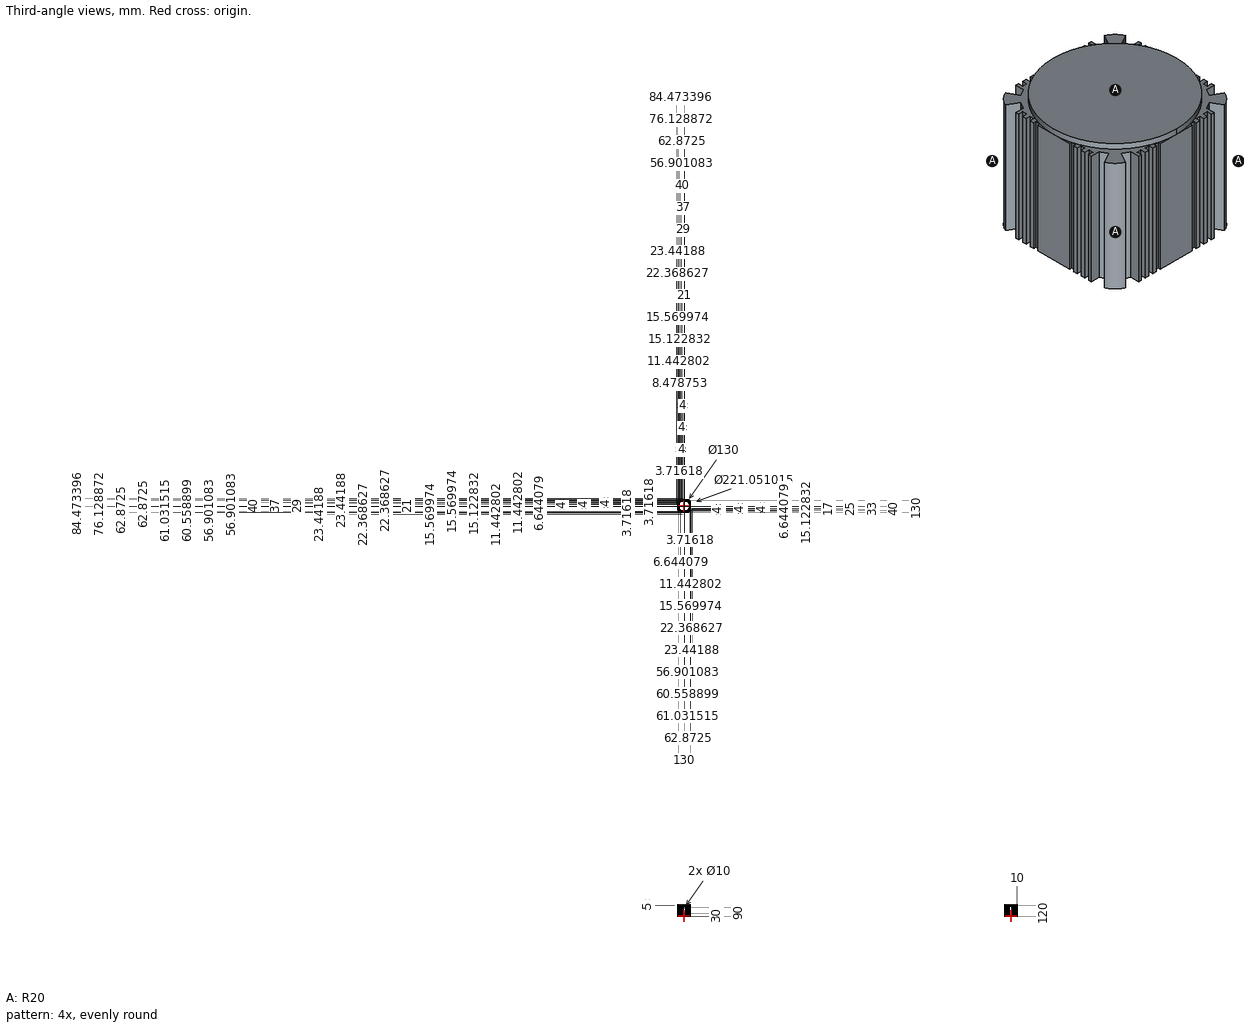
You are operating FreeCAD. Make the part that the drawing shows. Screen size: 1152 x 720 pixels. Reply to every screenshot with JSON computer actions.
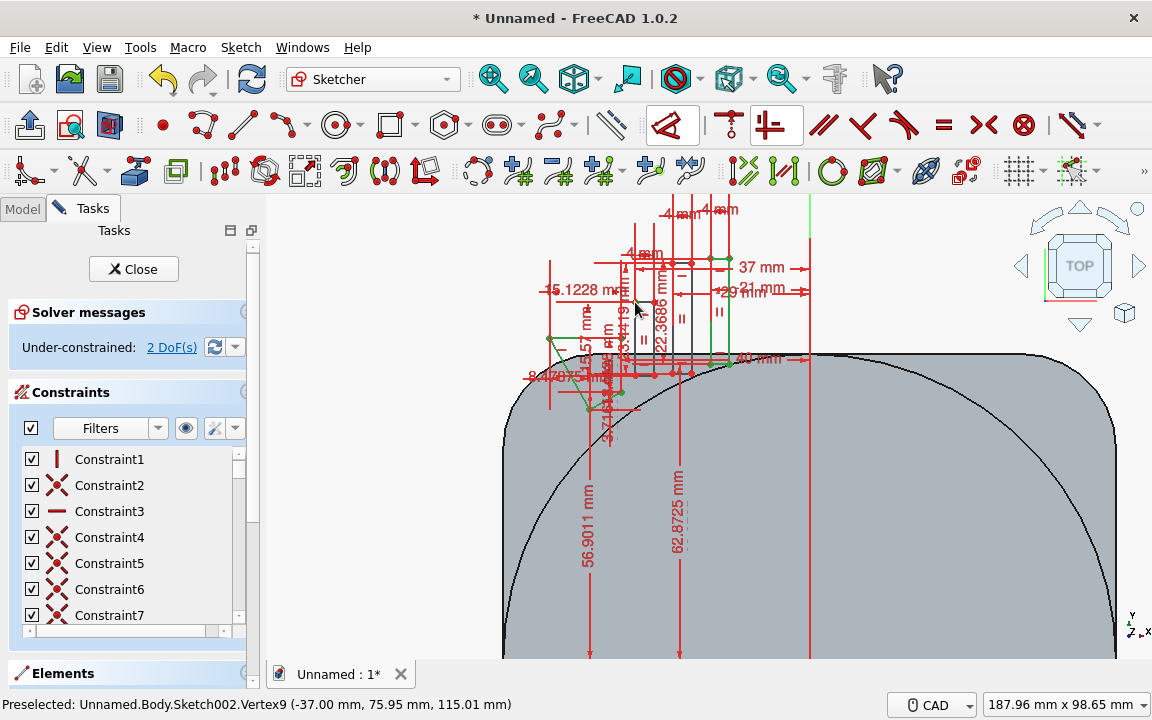
{"action": "left_click", "coordinate": [694, 126]}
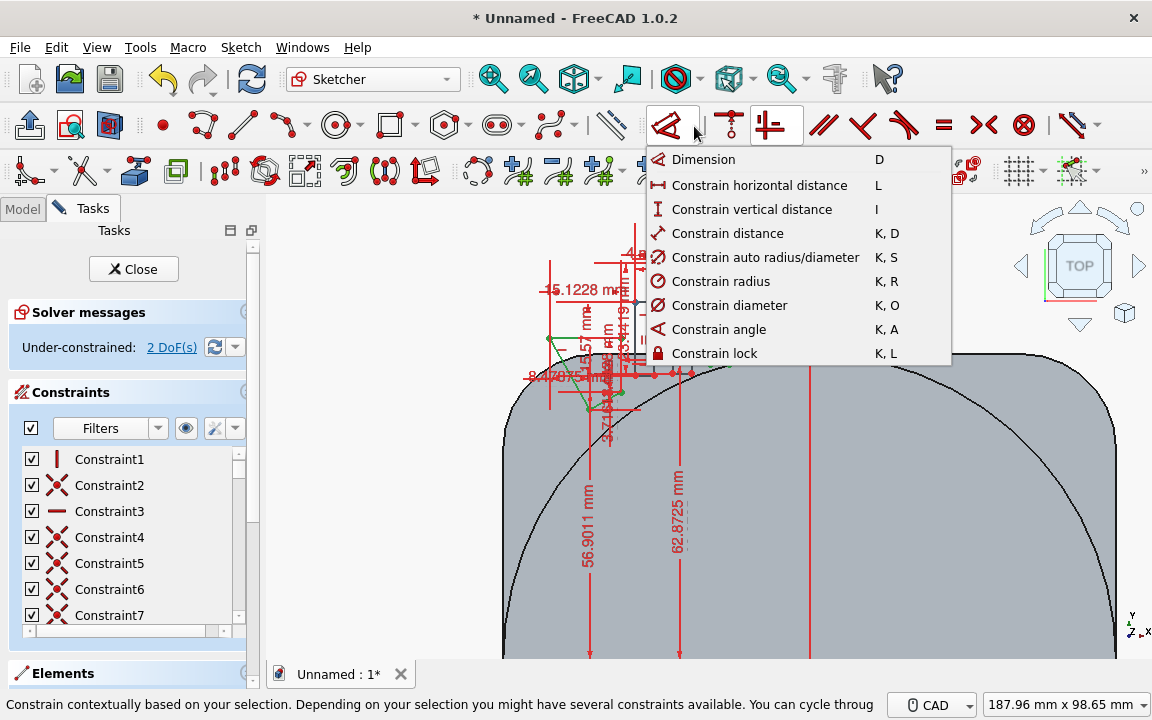
{"action": "left_click", "coordinate": [799, 209]}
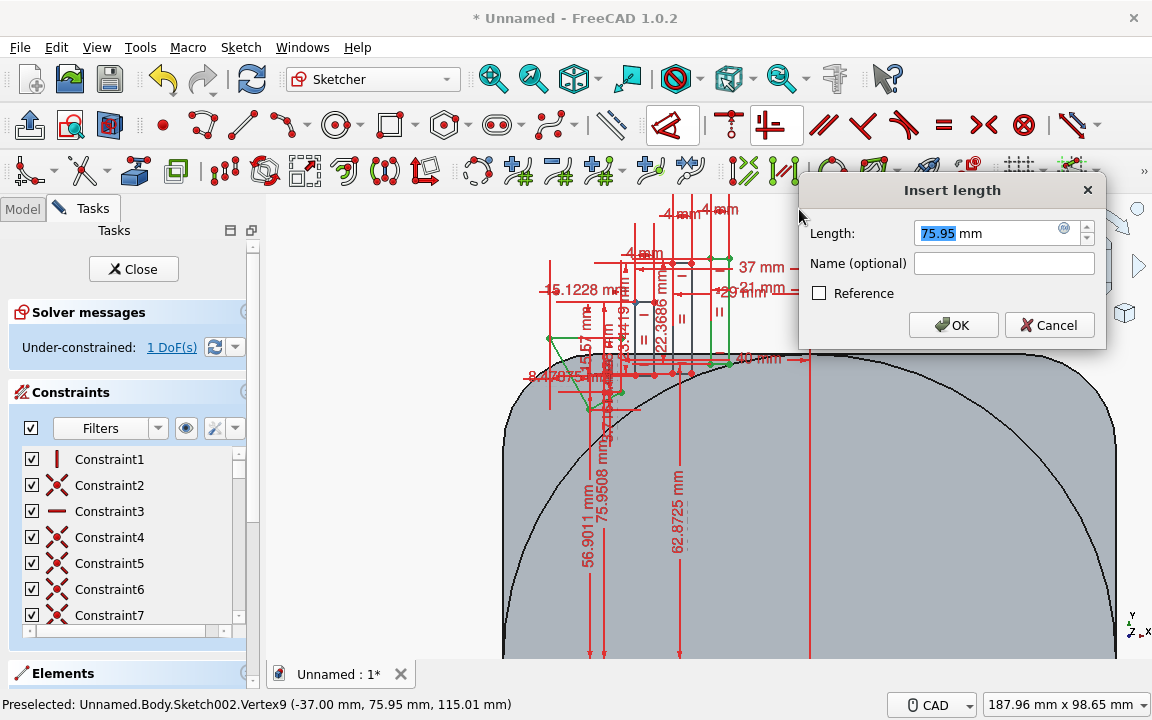
{"action": "type", "text": "76.128872"}
{"action": "key", "text": "Return"}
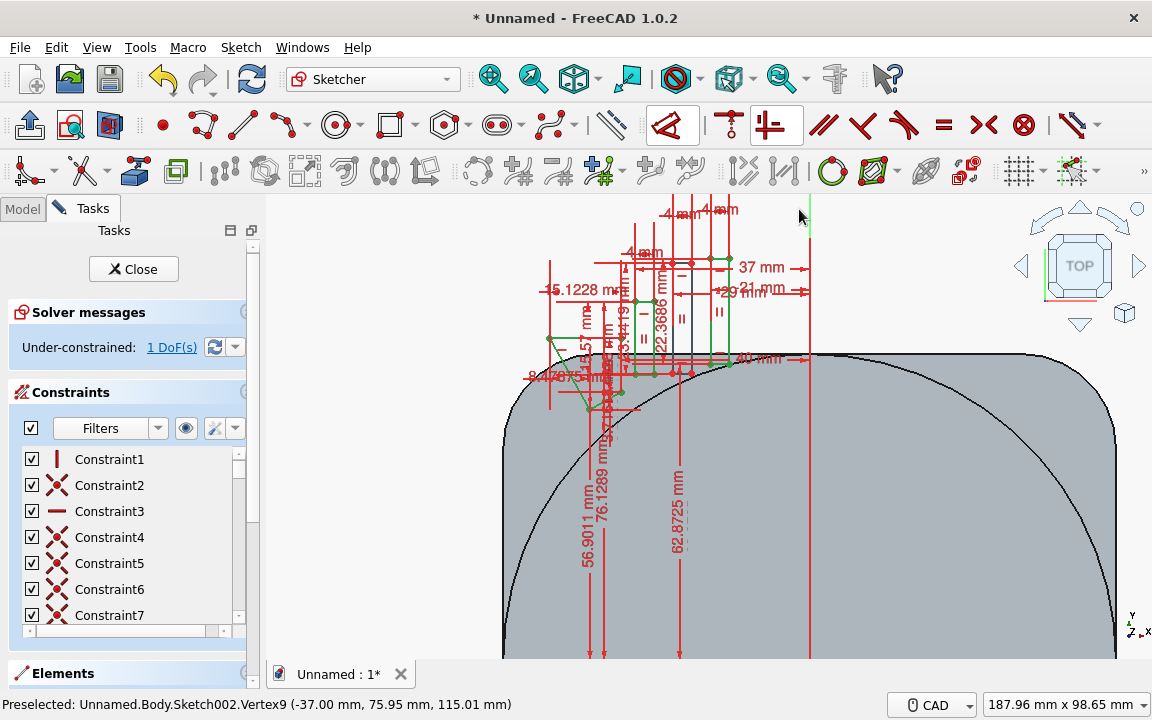
{"action": "left_click", "coordinate": [673, 263]}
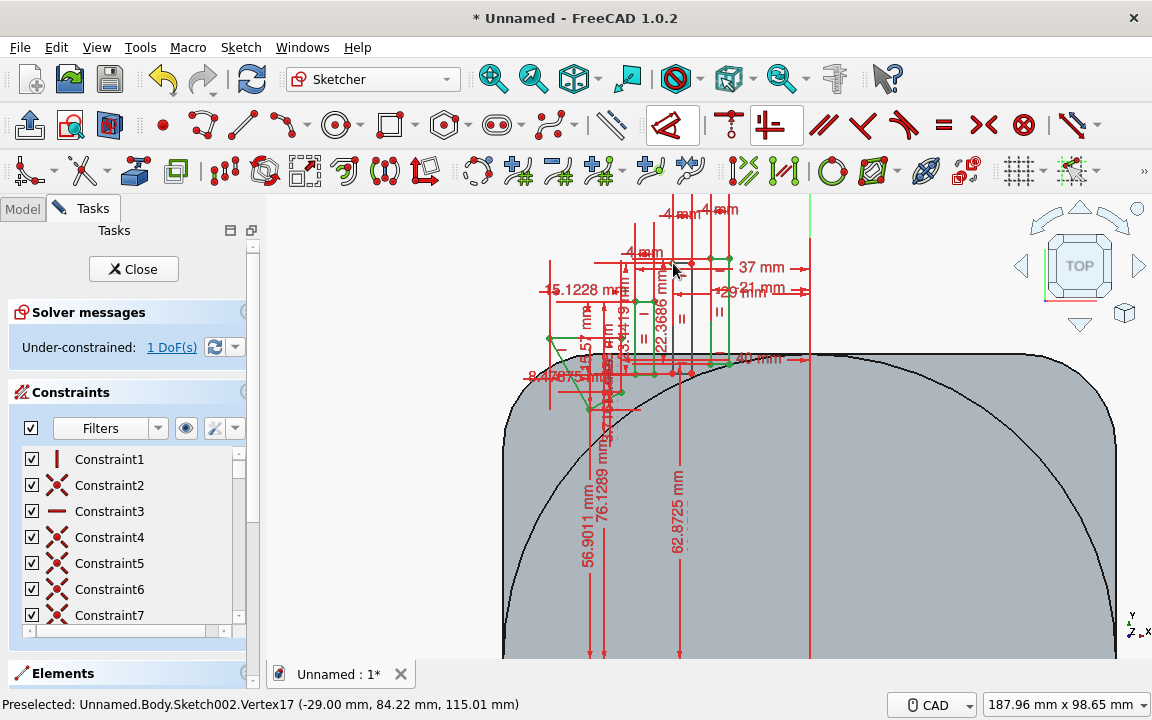
{"action": "left_click", "coordinate": [694, 126]}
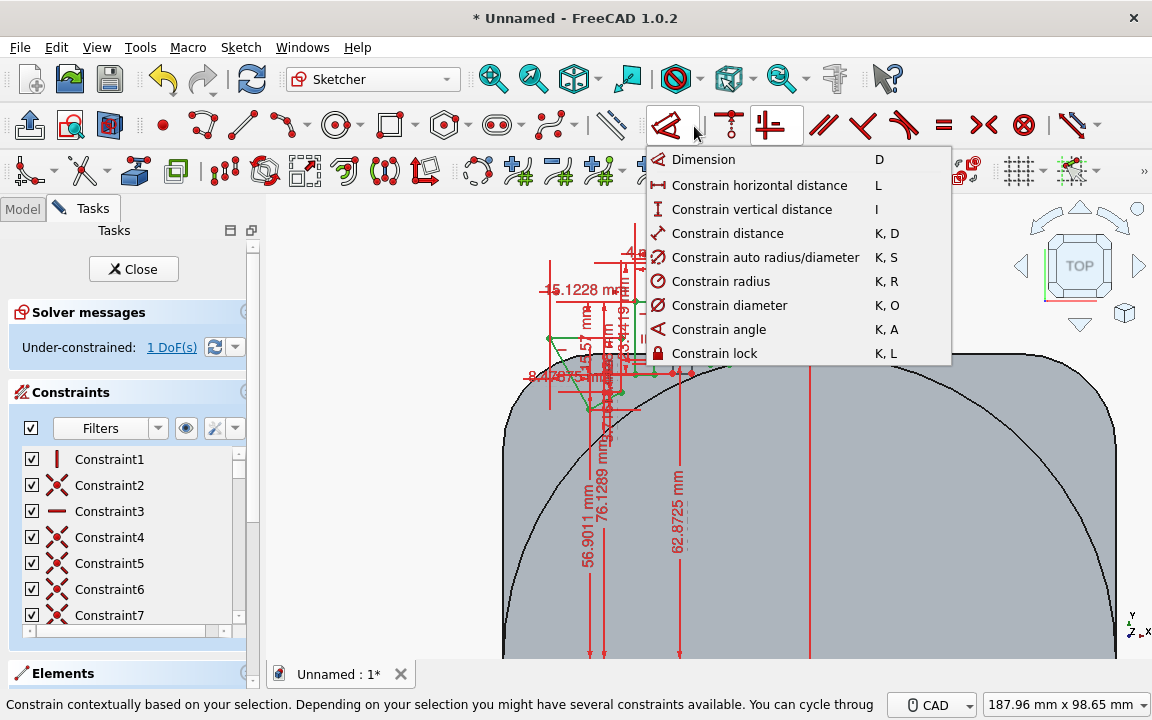
{"action": "left_click", "coordinate": [799, 209]}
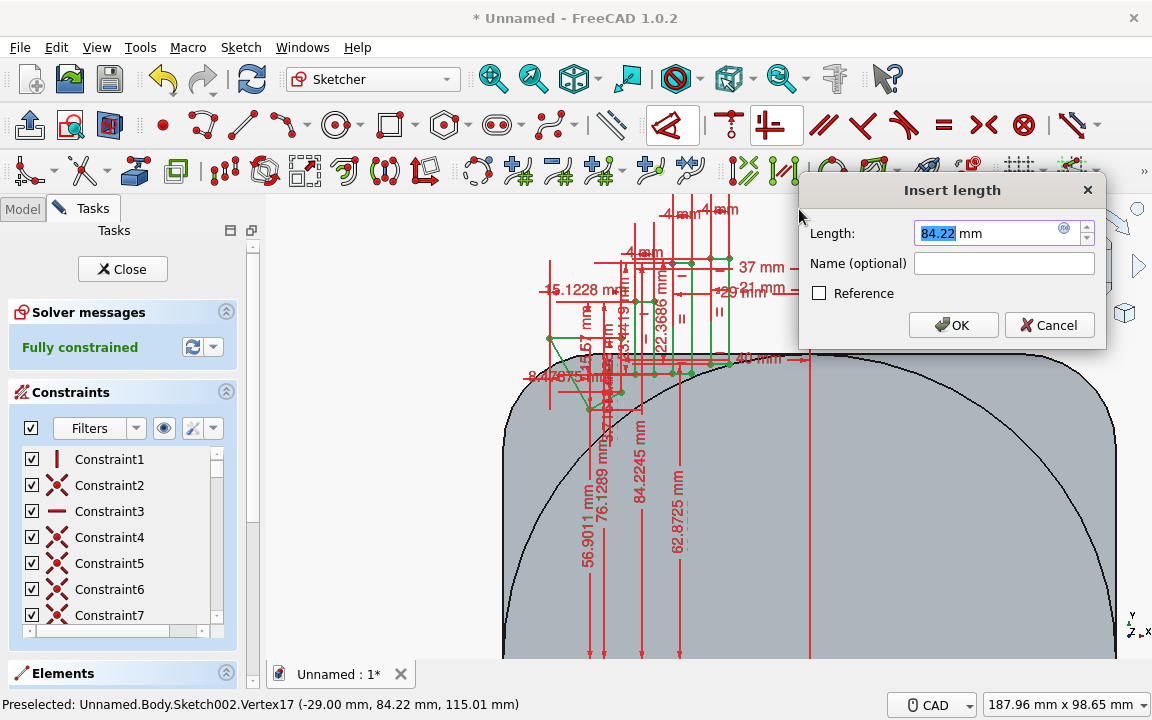
{"action": "type", "text": "84.473396"}
{"action": "key", "text": "Return"}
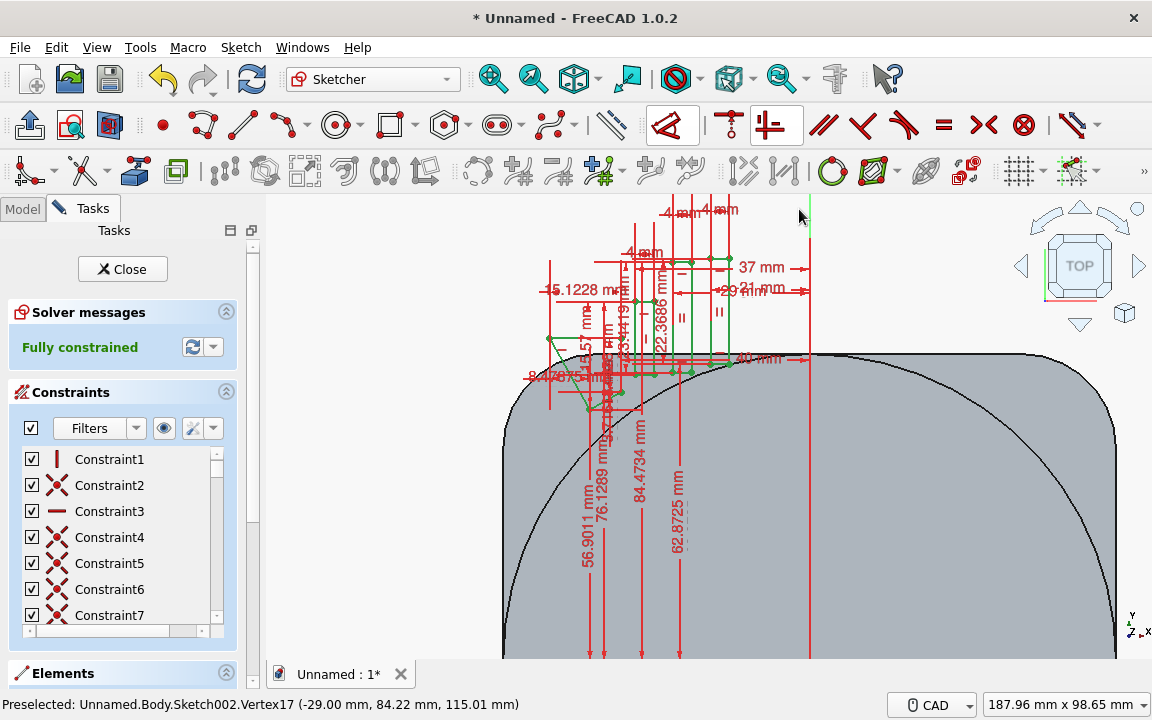
{"action": "left_click", "coordinate": [123, 269]}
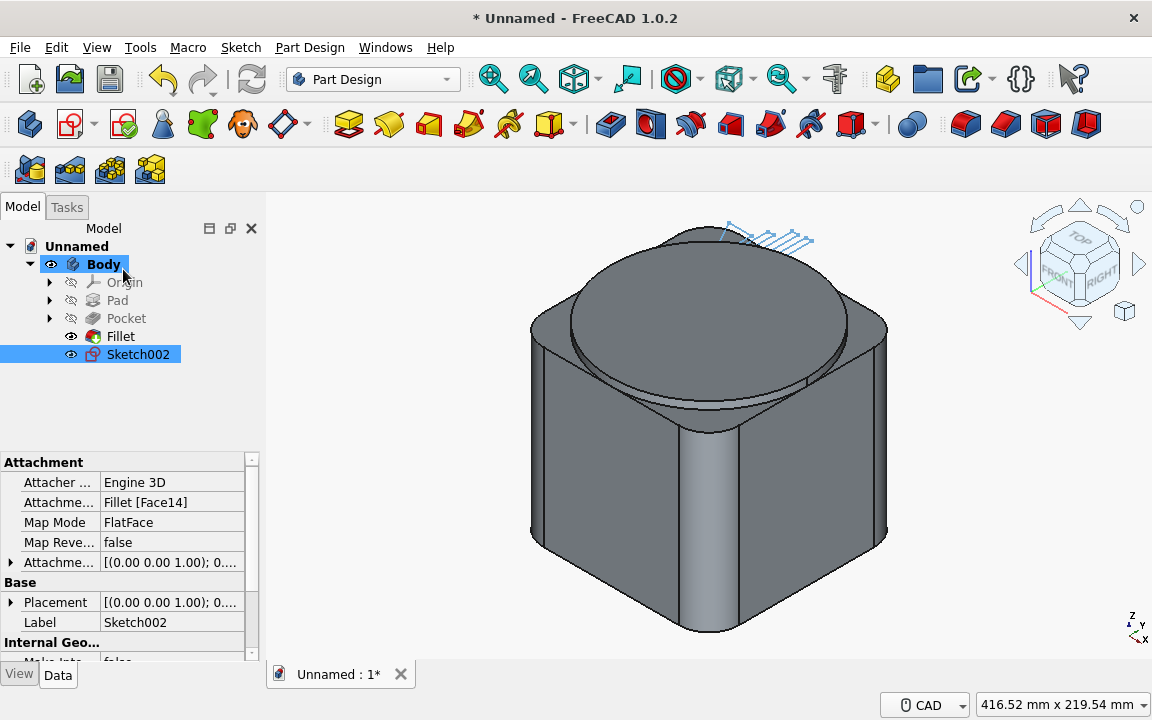
{"action": "left_click", "coordinate": [612, 124]}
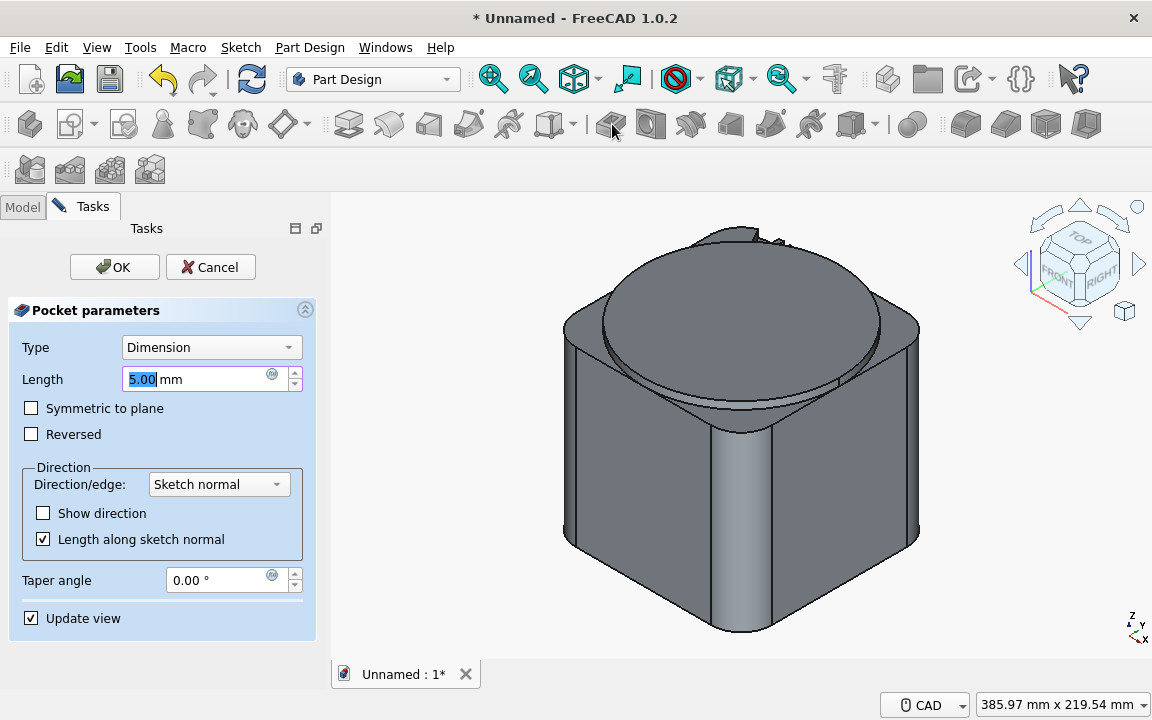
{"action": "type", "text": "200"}
{"action": "key", "text": "Tab"}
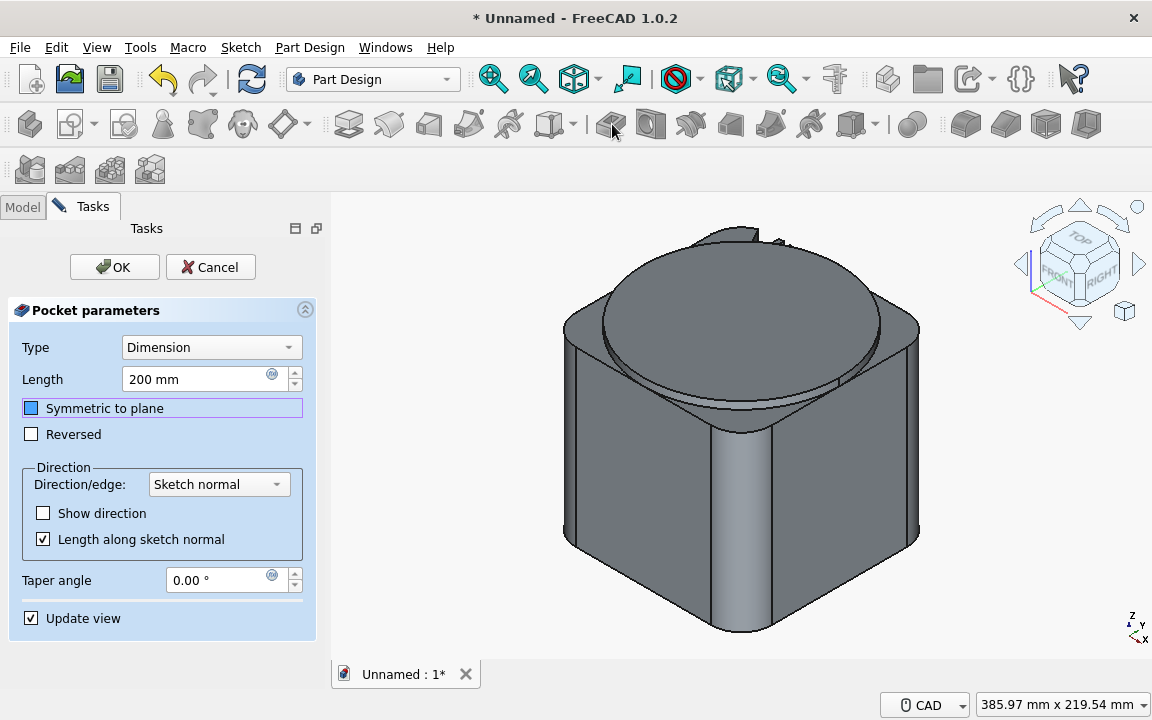
{"action": "left_click", "coordinate": [115, 267]}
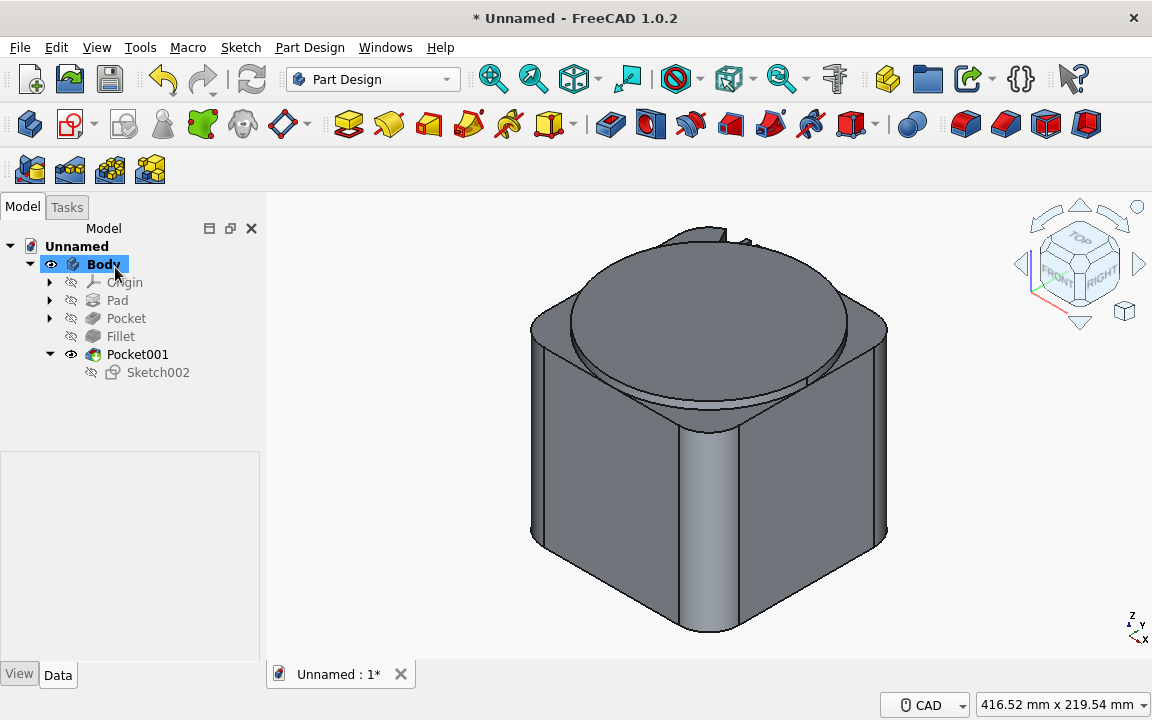
{"action": "left_click", "coordinate": [116, 354]}